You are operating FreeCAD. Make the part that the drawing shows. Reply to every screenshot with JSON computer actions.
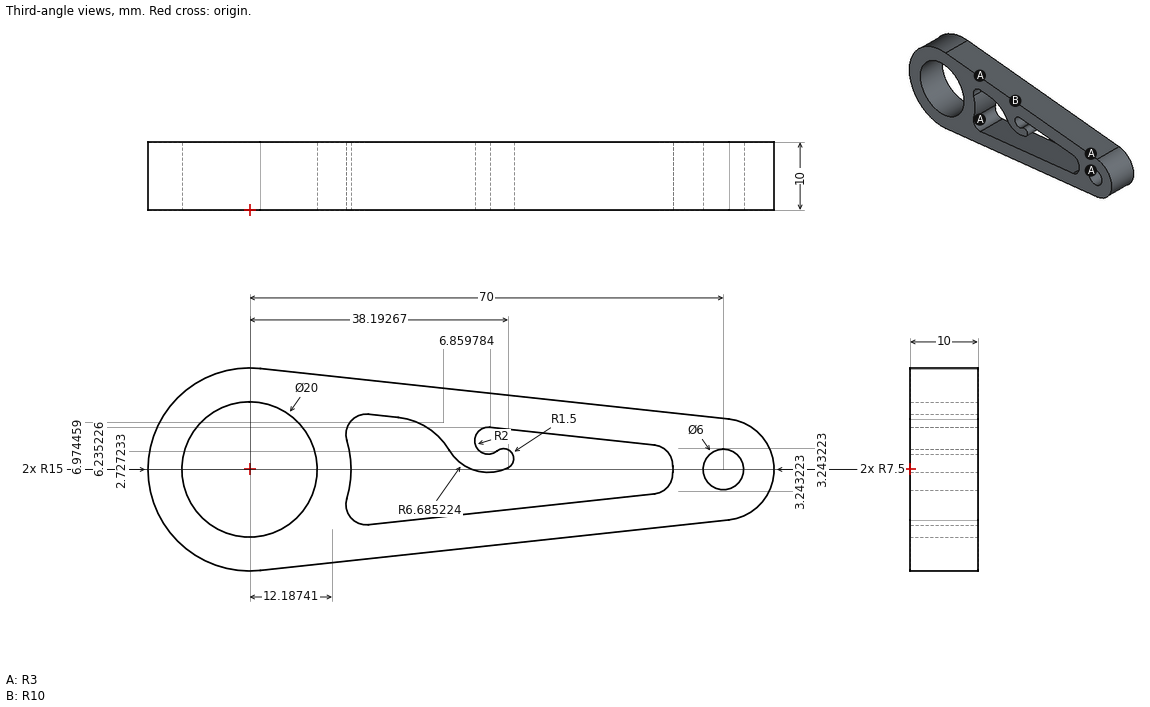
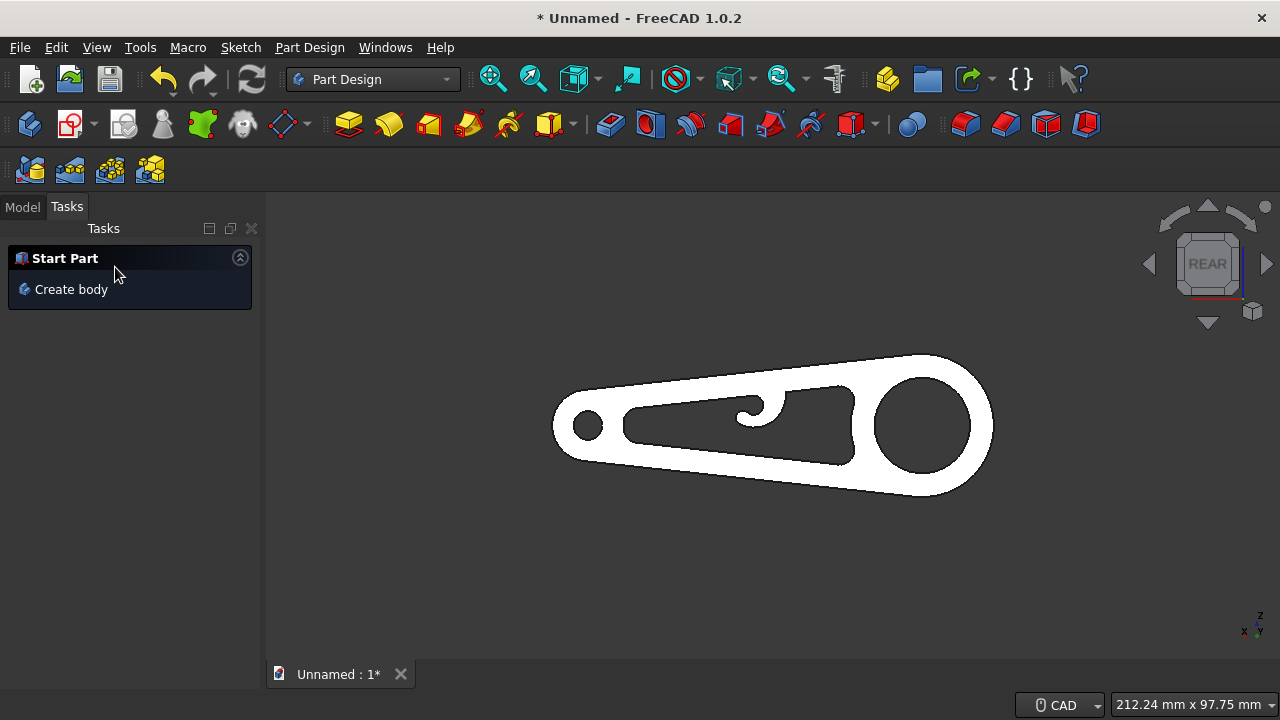
{"action": "left_click", "coordinate": [494, 80]}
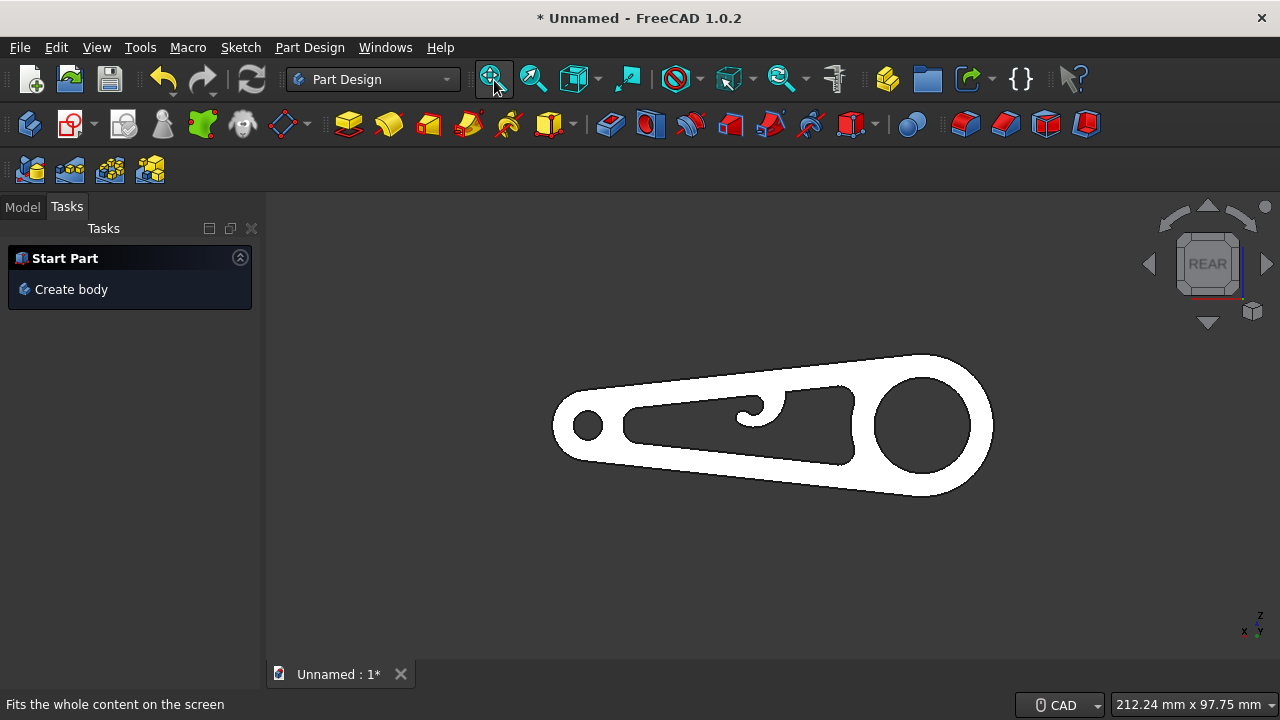
{"action": "key", "text": "0"}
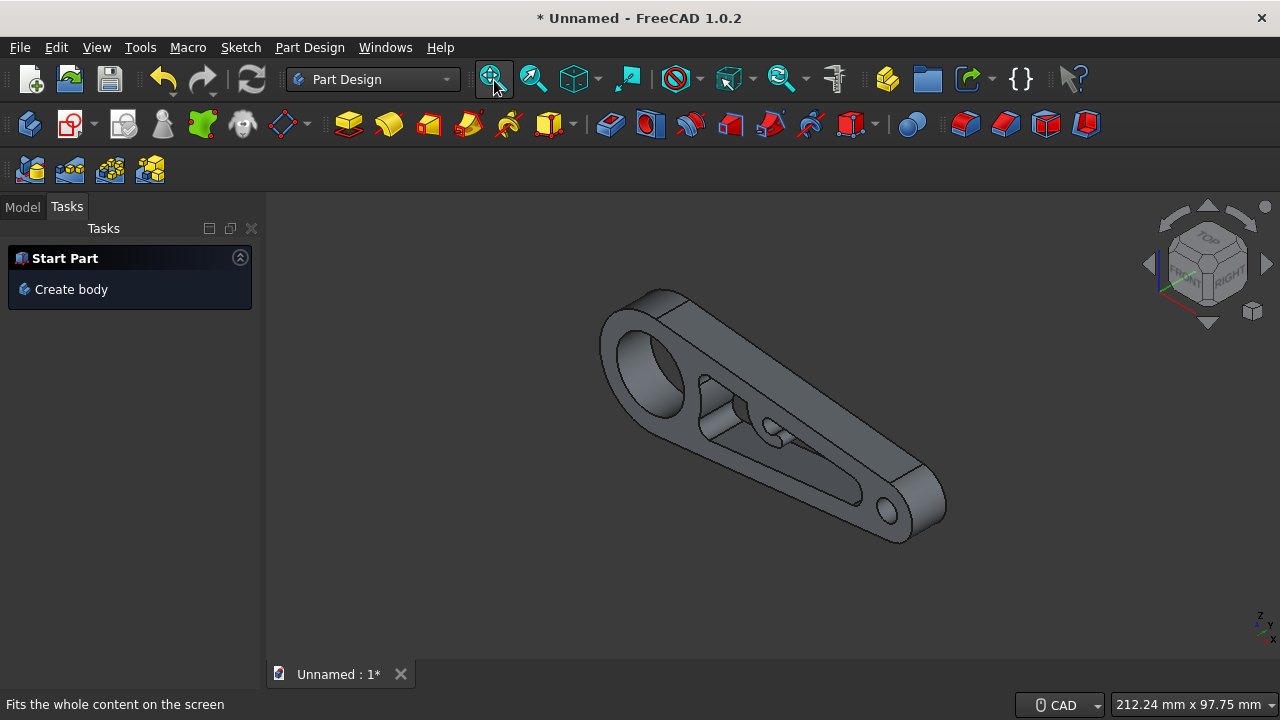
{"action": "key", "text": "2"}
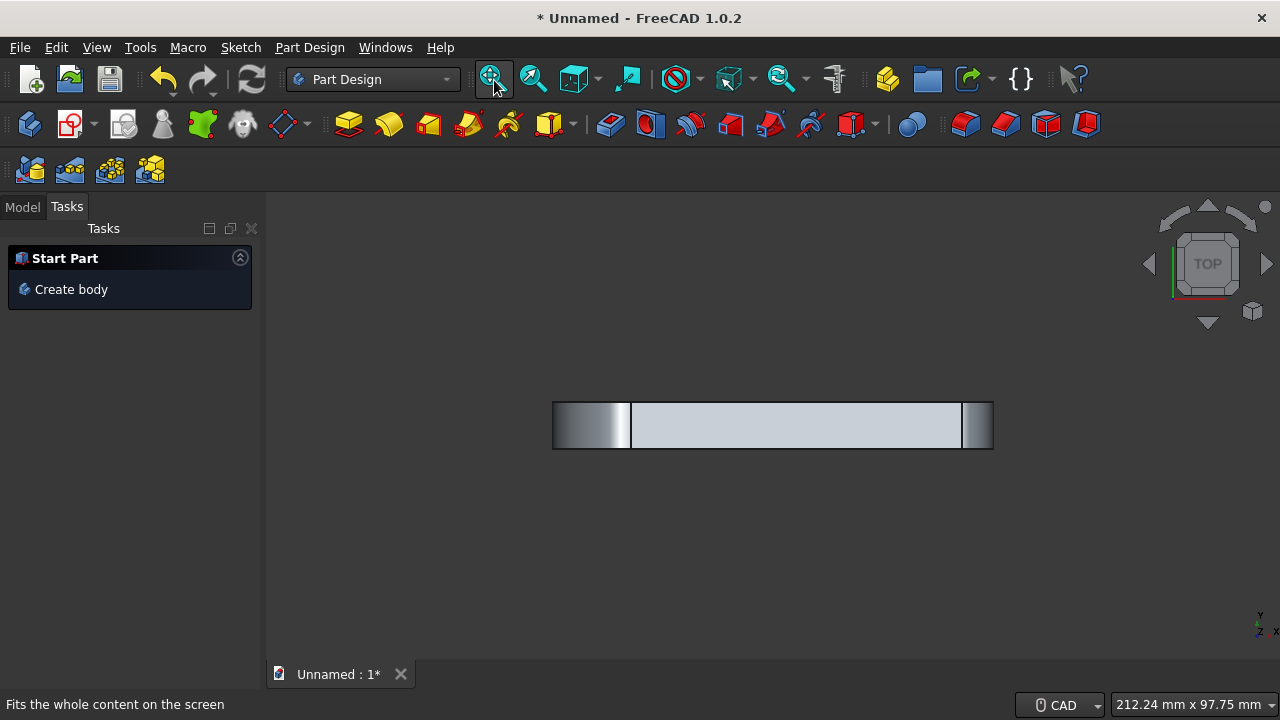
{"action": "left_click", "coordinate": [494, 80]}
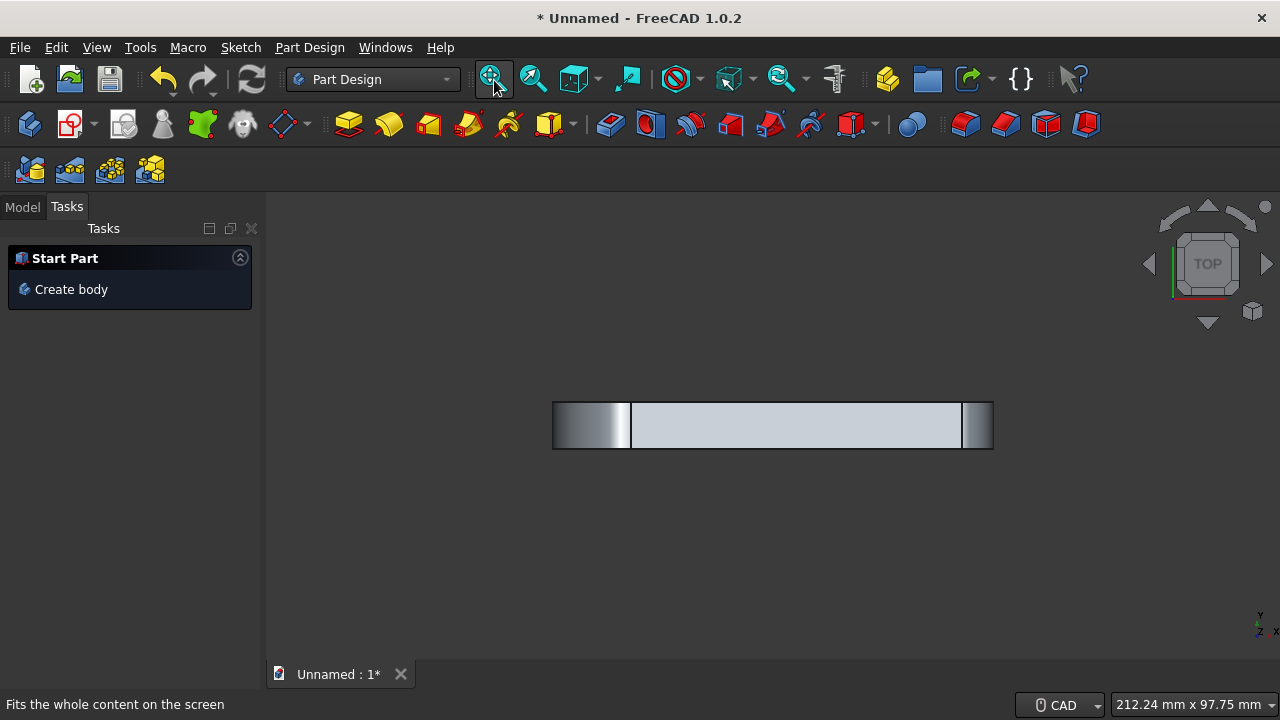
{"action": "key", "text": "1"}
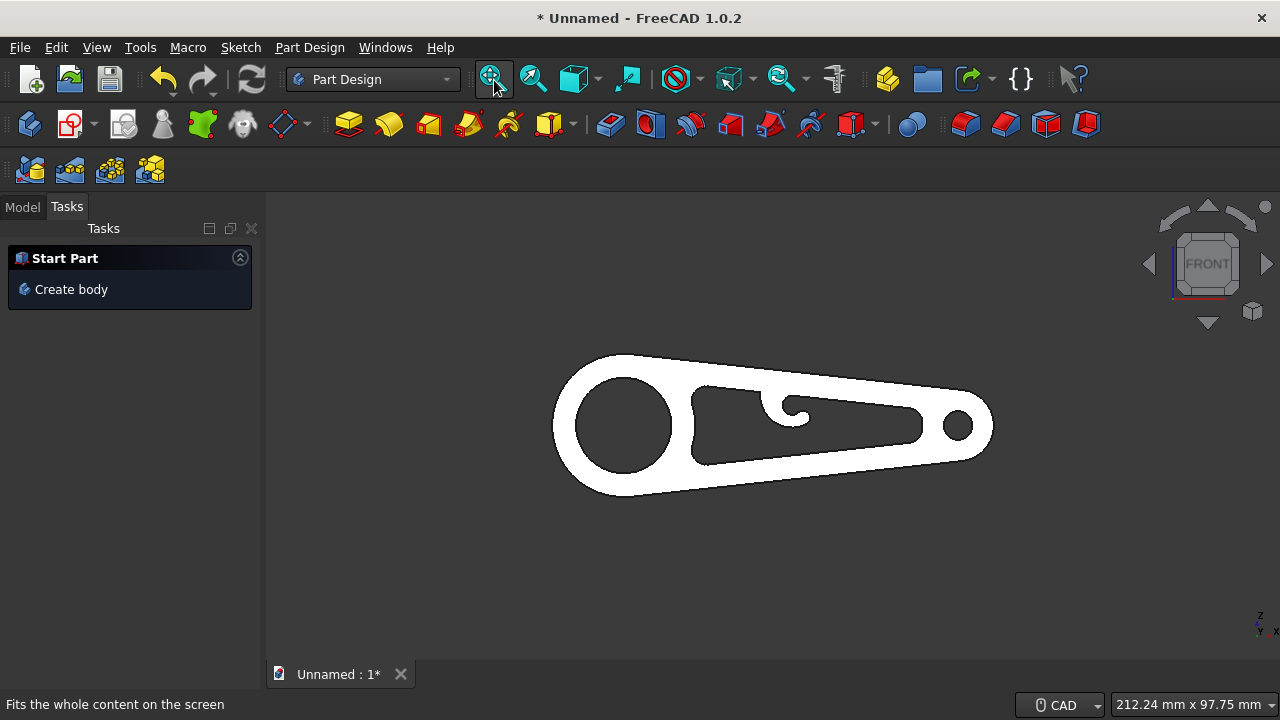
{"action": "left_click", "coordinate": [494, 80]}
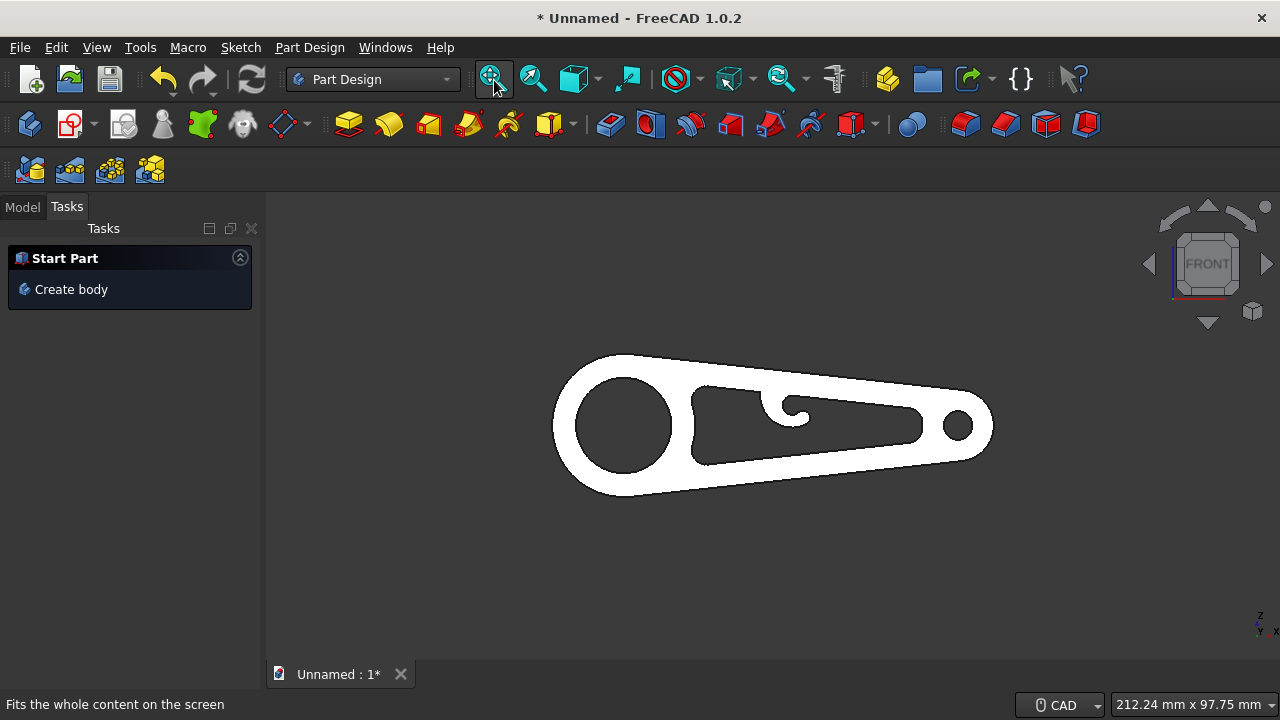
{"action": "key", "text": "3"}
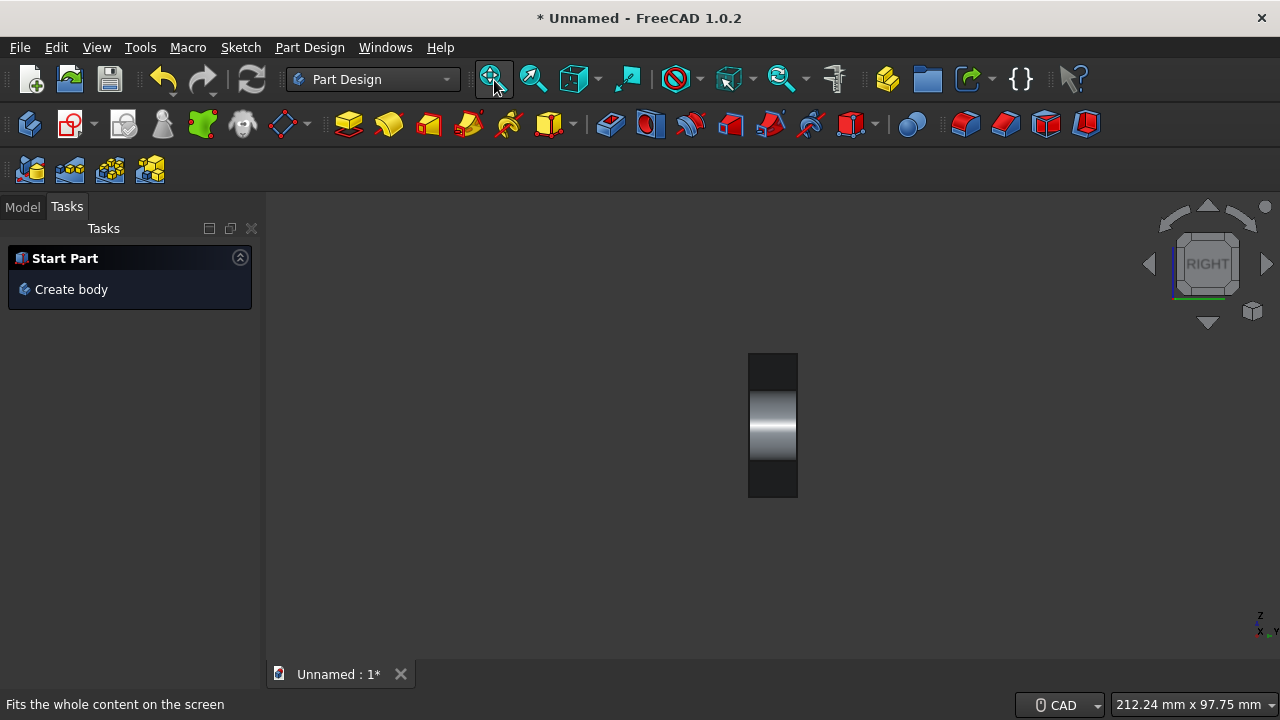
{"action": "left_click", "coordinate": [494, 80]}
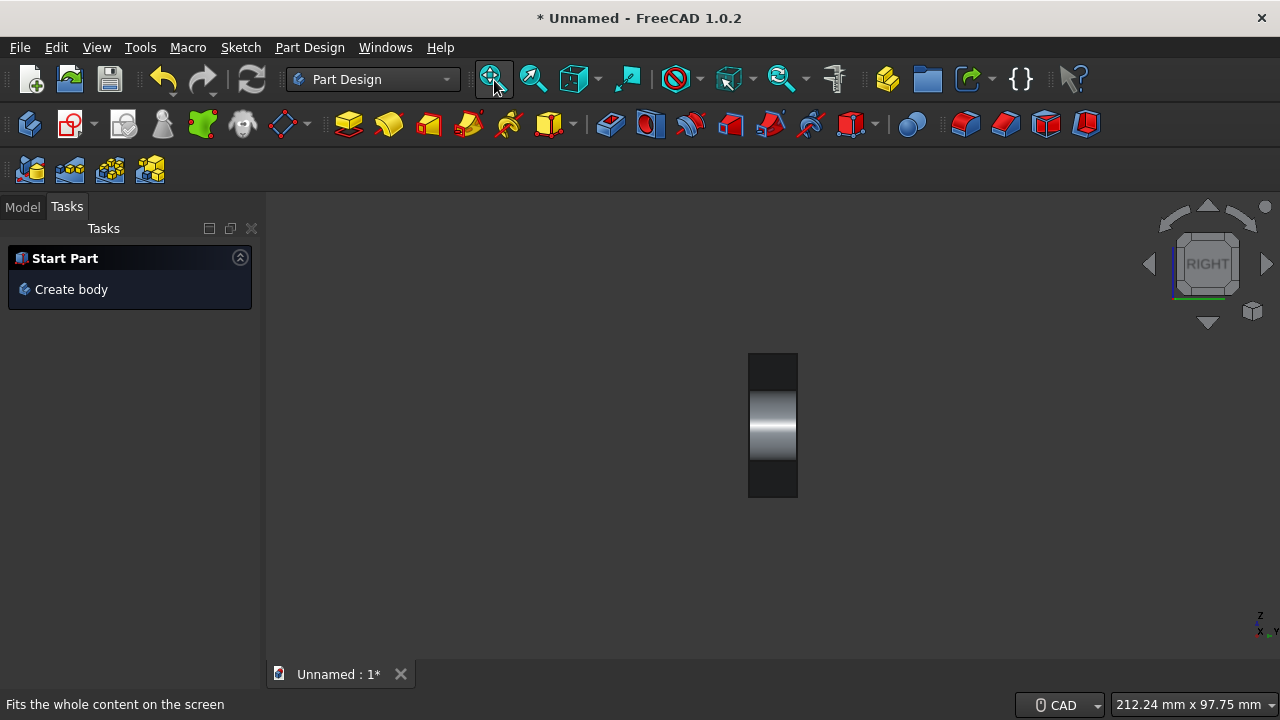
{"action": "key", "text": "5"}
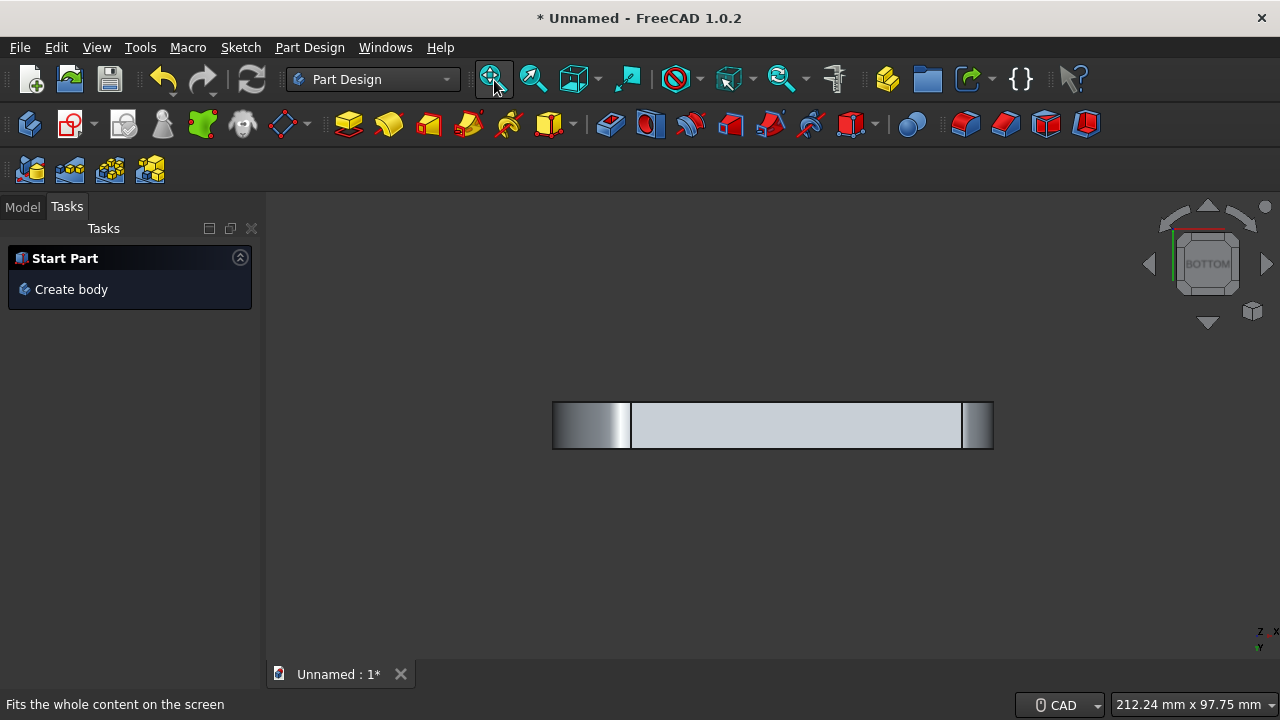
{"action": "left_click", "coordinate": [494, 80]}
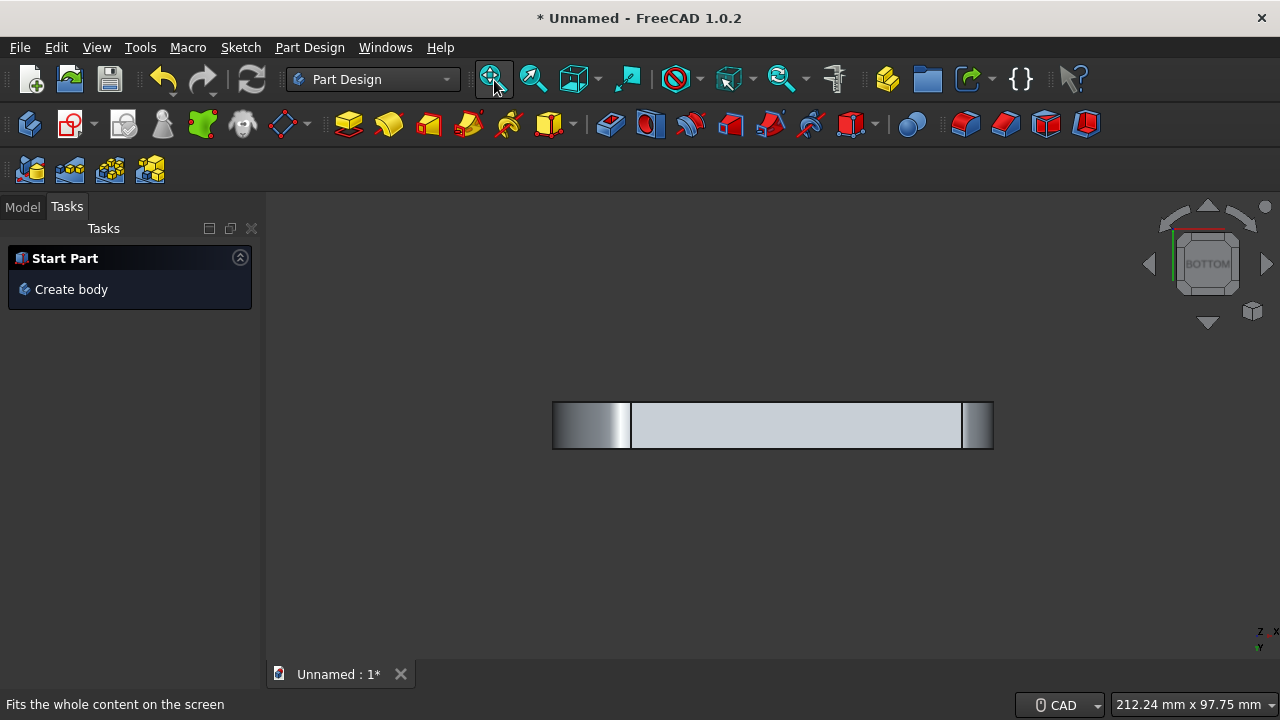
{"action": "key", "text": "4"}